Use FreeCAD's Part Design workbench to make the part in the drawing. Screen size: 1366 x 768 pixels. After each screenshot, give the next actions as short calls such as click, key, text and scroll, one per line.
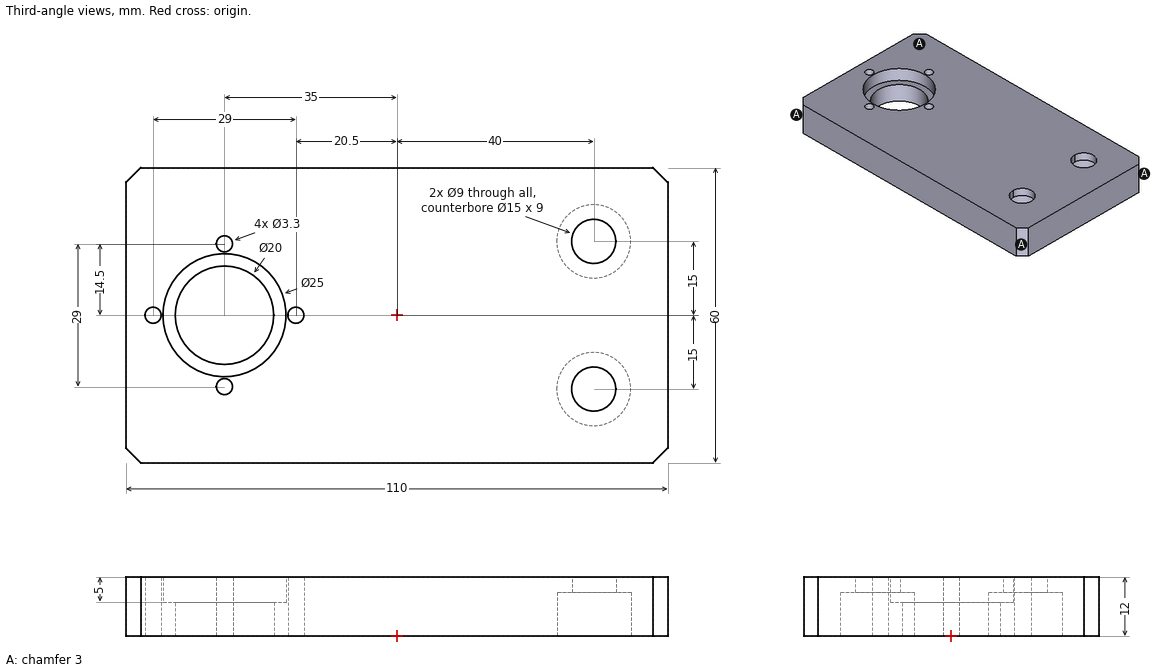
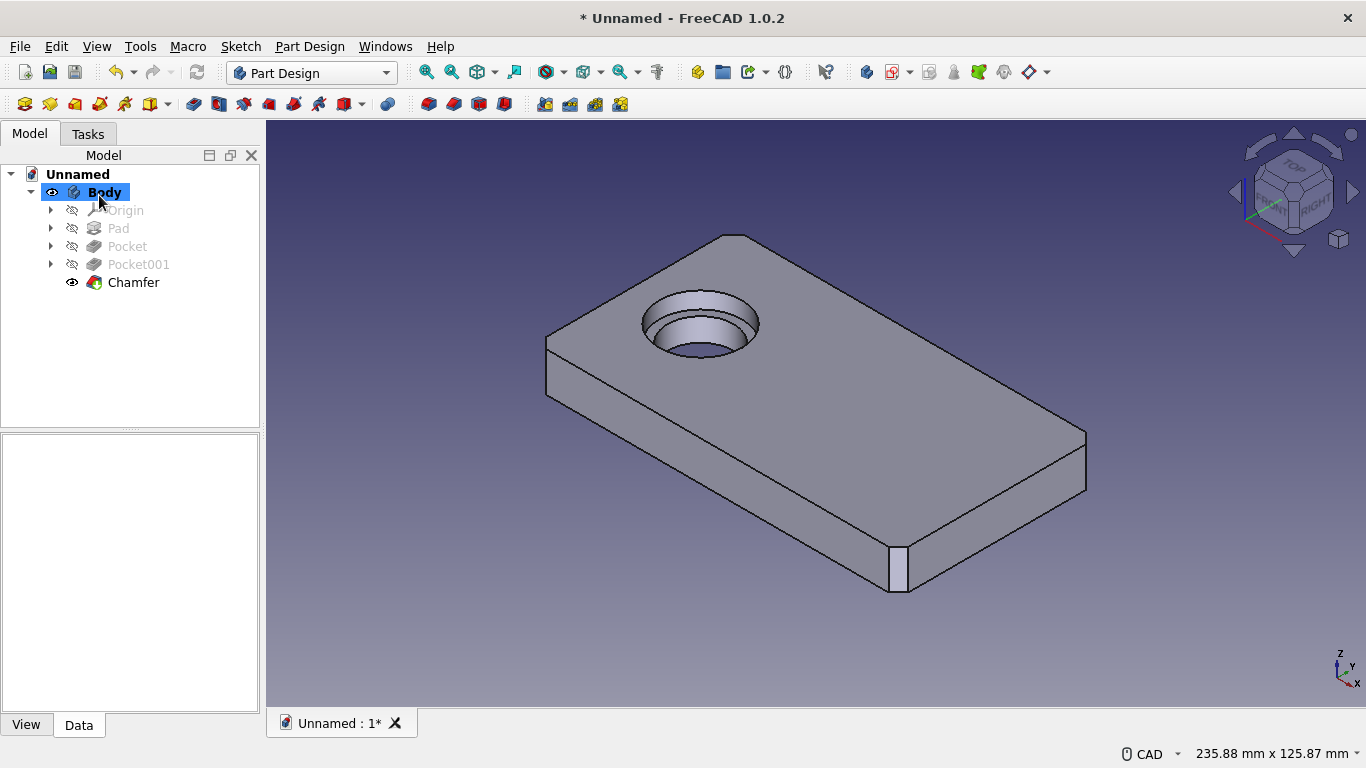
click(868, 420)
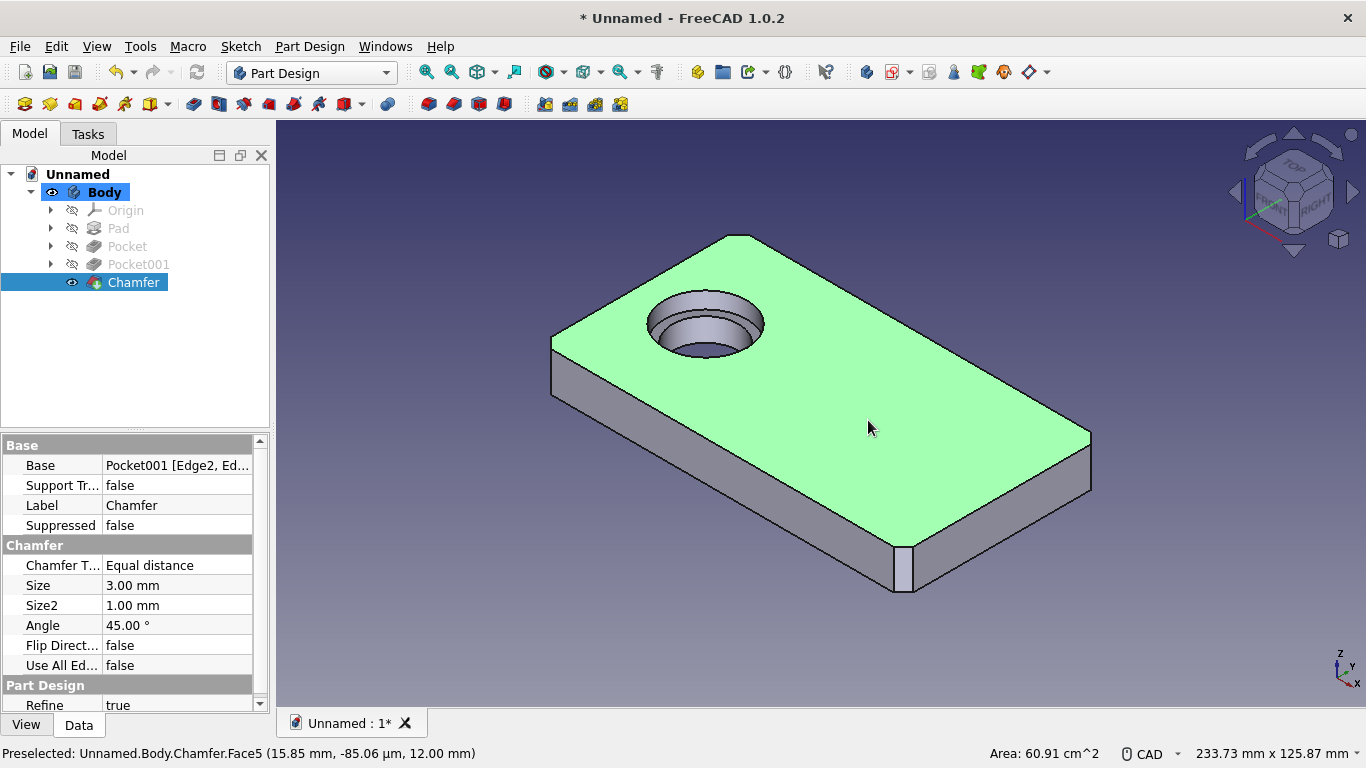
click(892, 72)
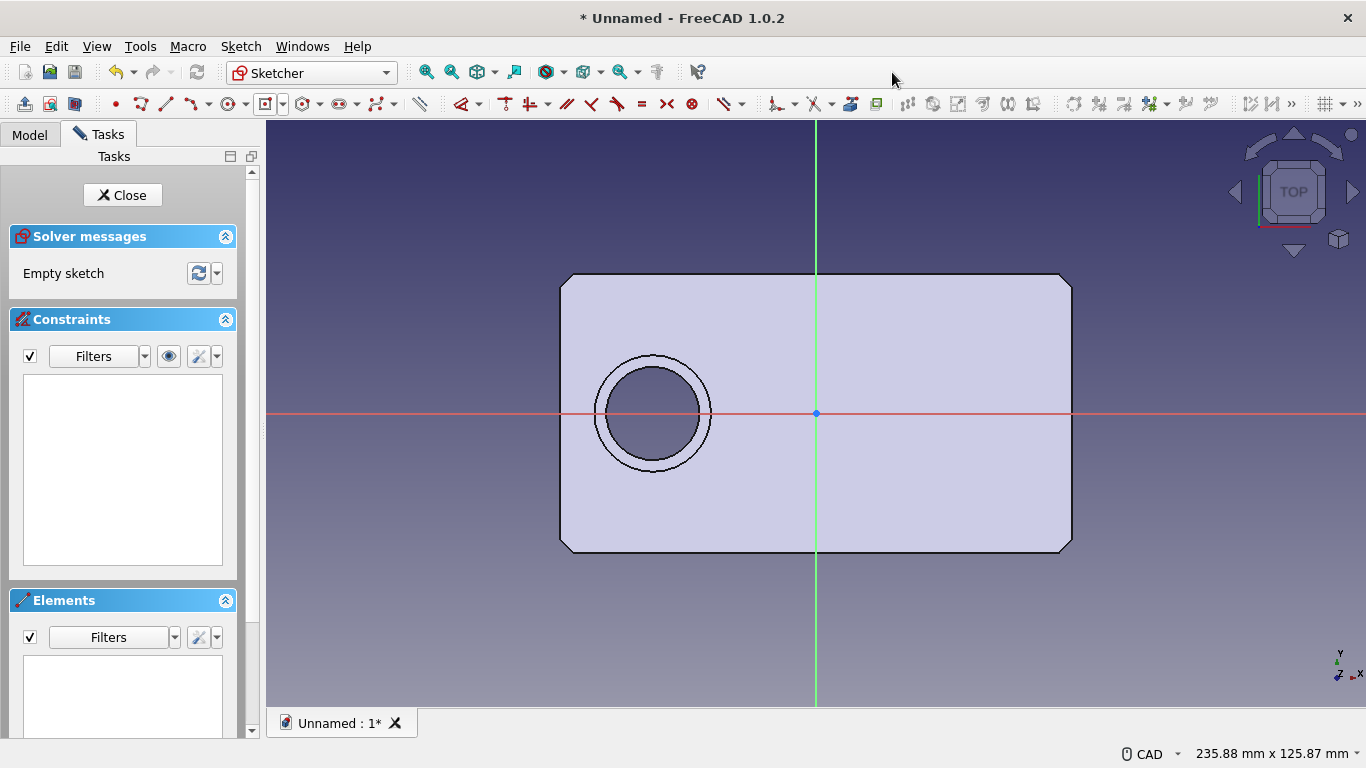
scroll(667, 414, up, 5)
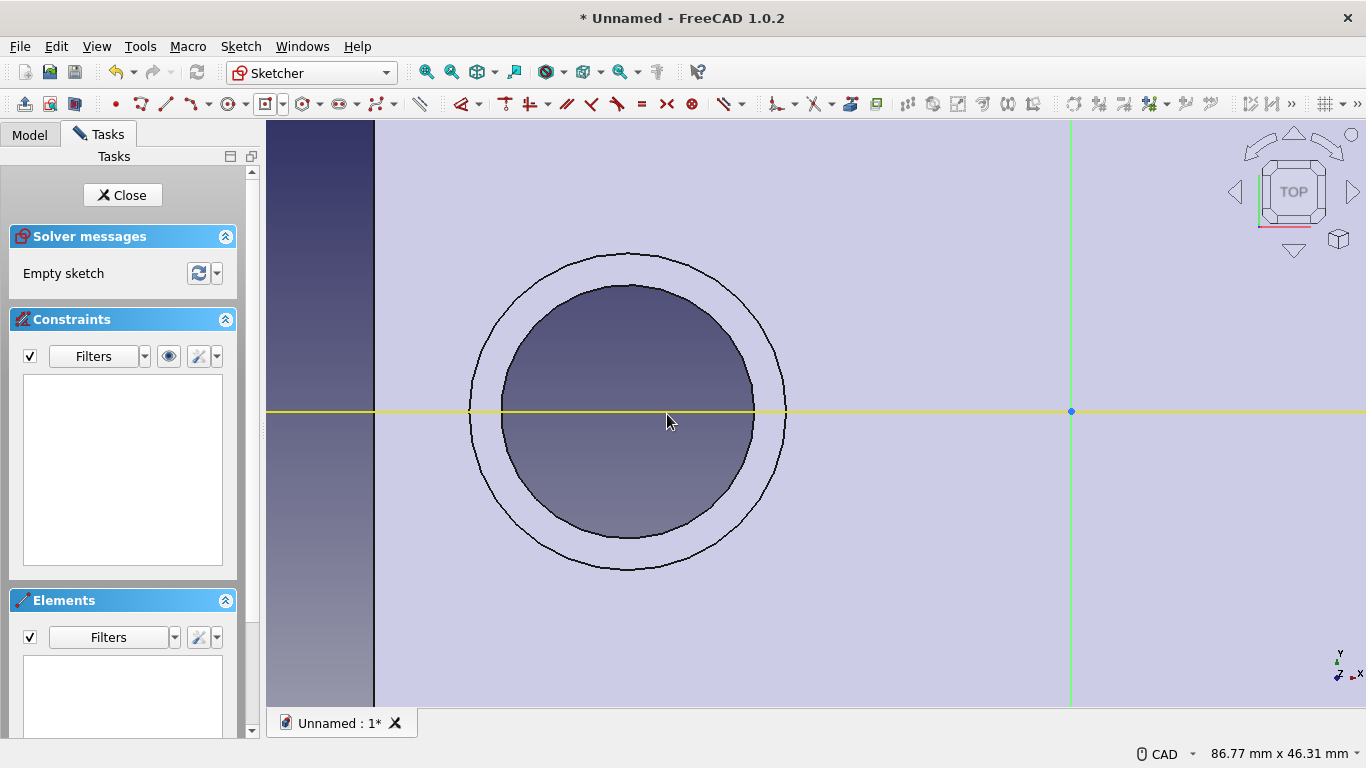
key(g)
key(c)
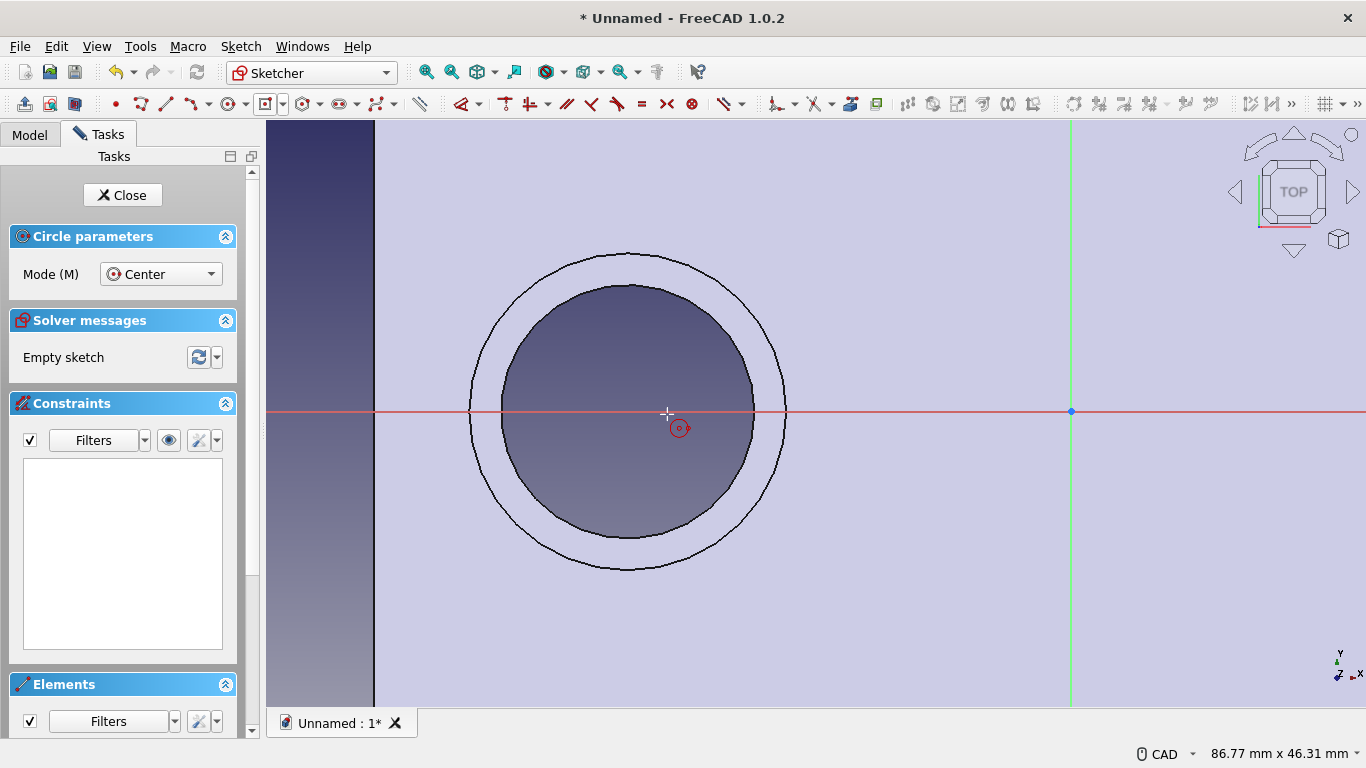
click(628, 228)
click(643, 213)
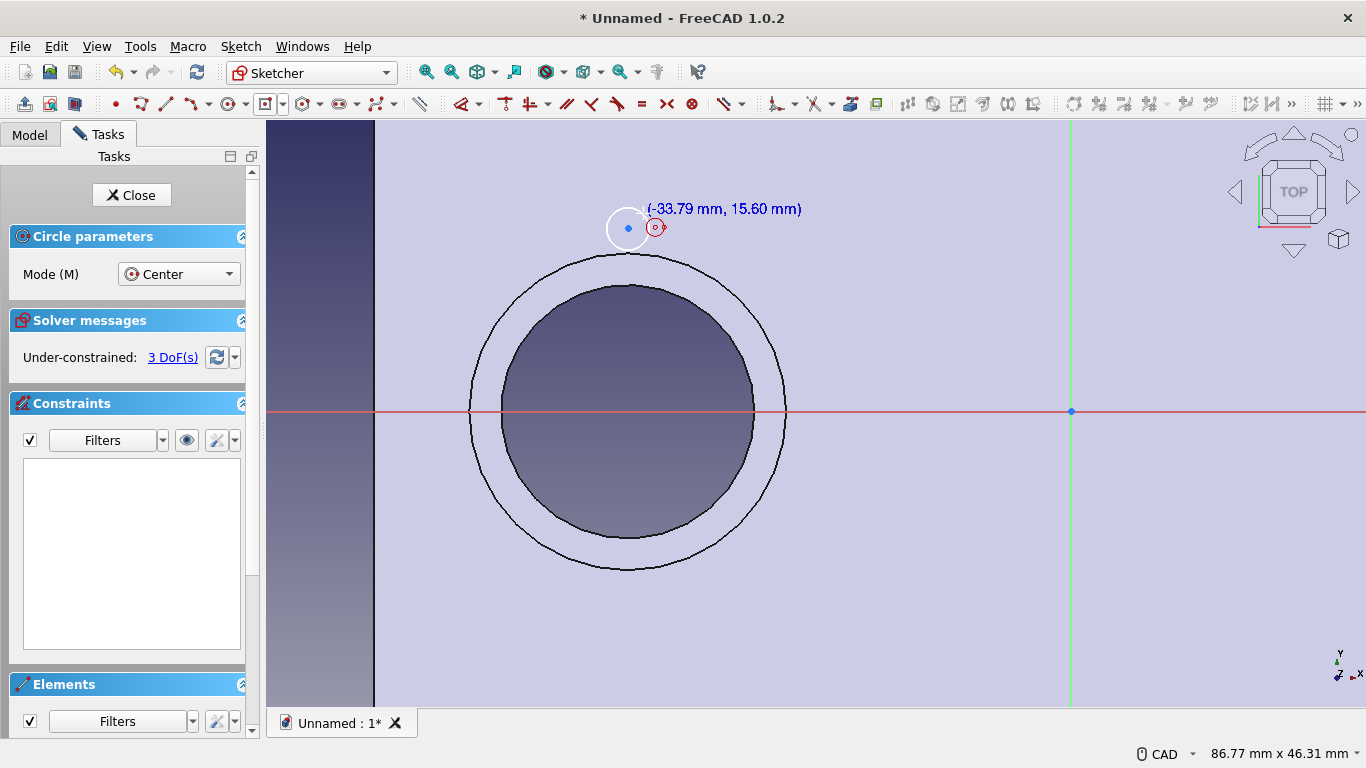
click(812, 412)
click(826, 397)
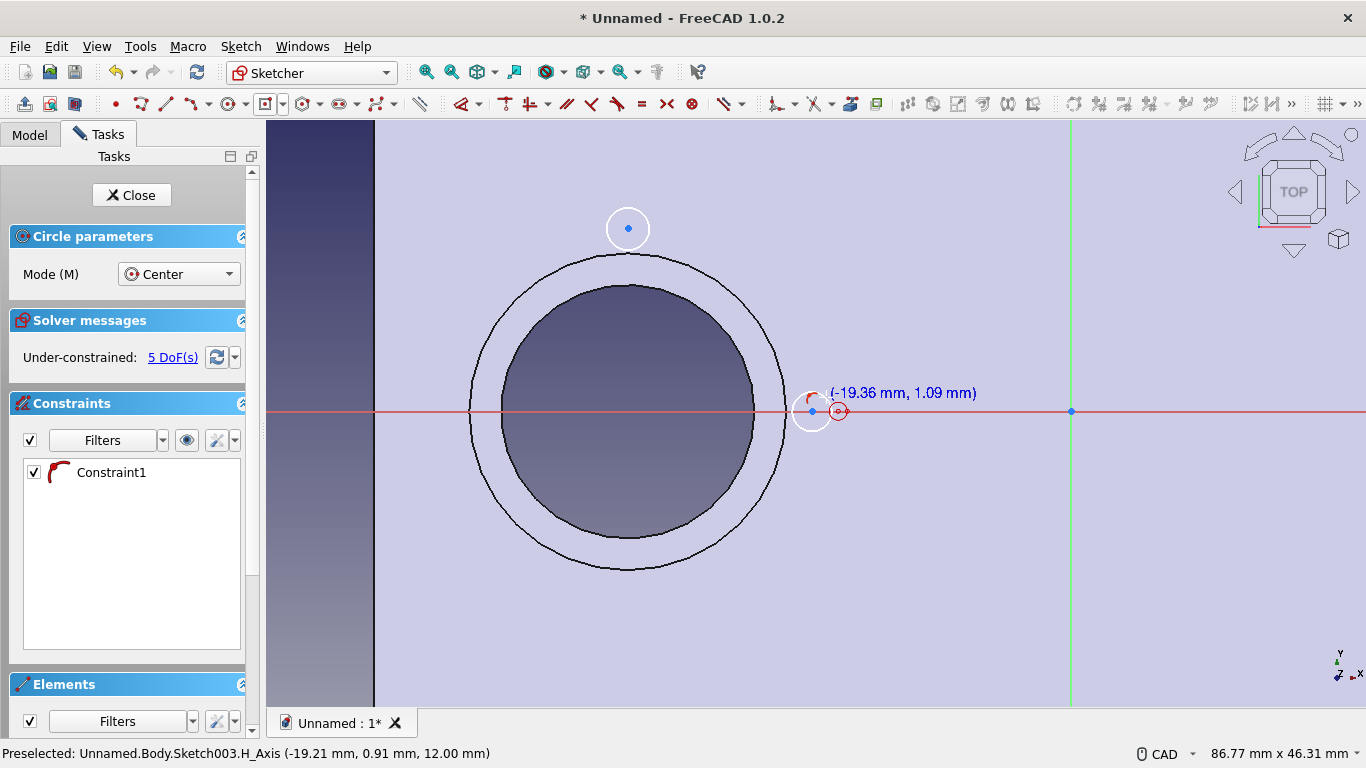
click(444, 412)
click(459, 397)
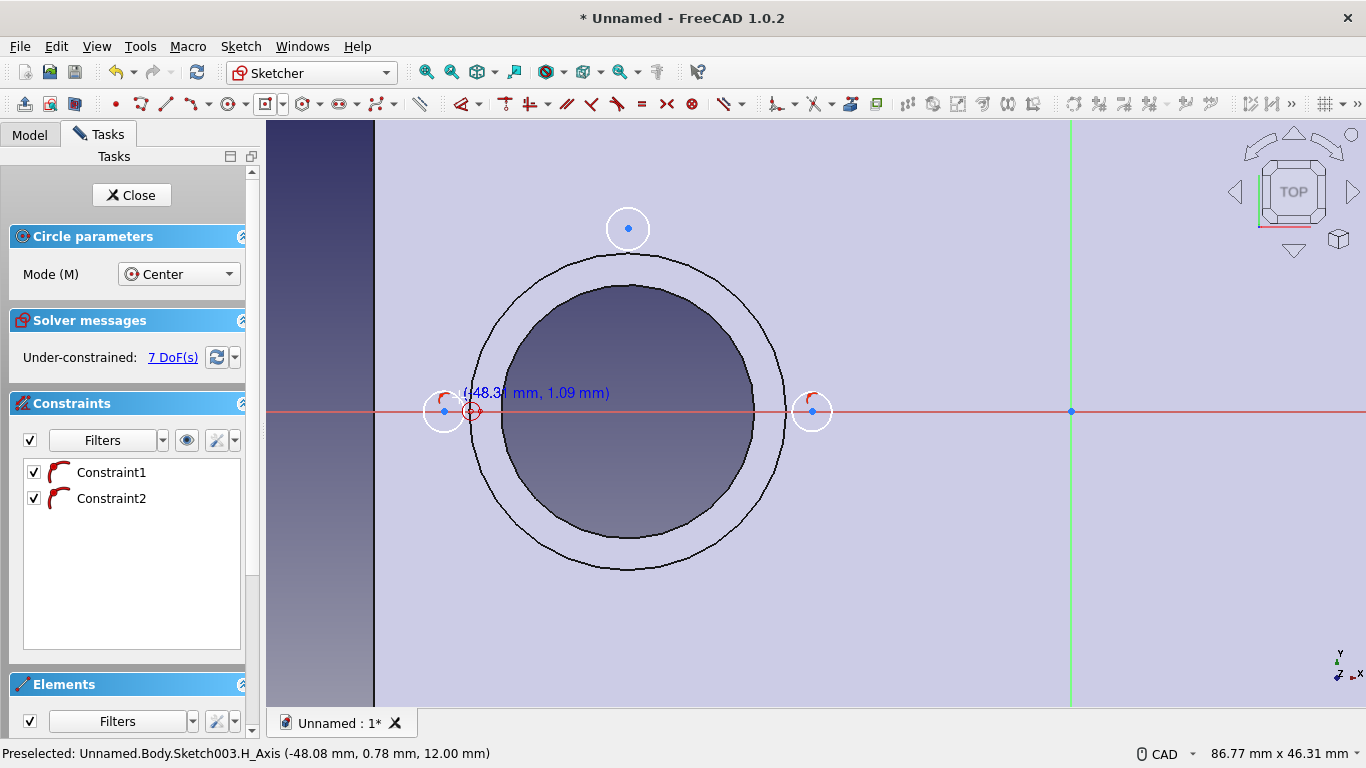
click(628, 596)
click(643, 581)
key(Escape)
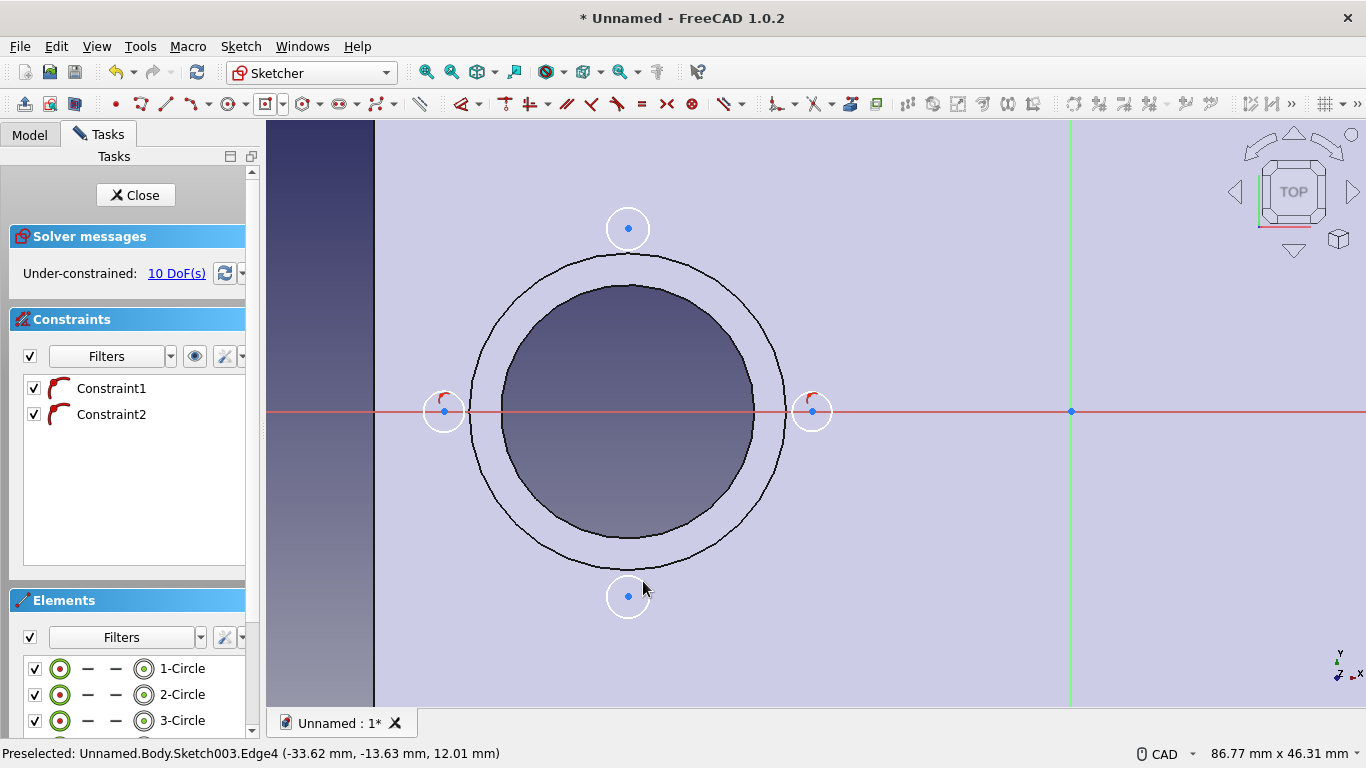
click(643, 214)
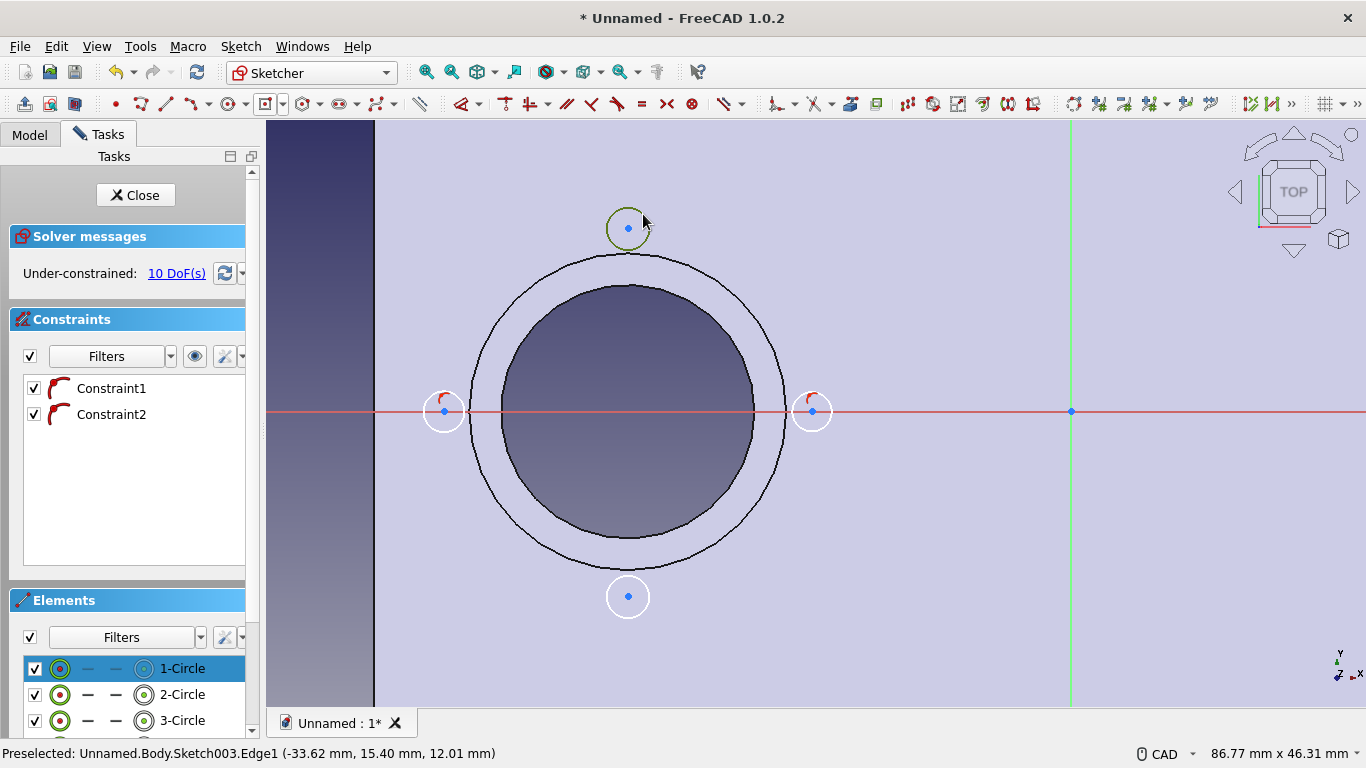
click(826, 398)